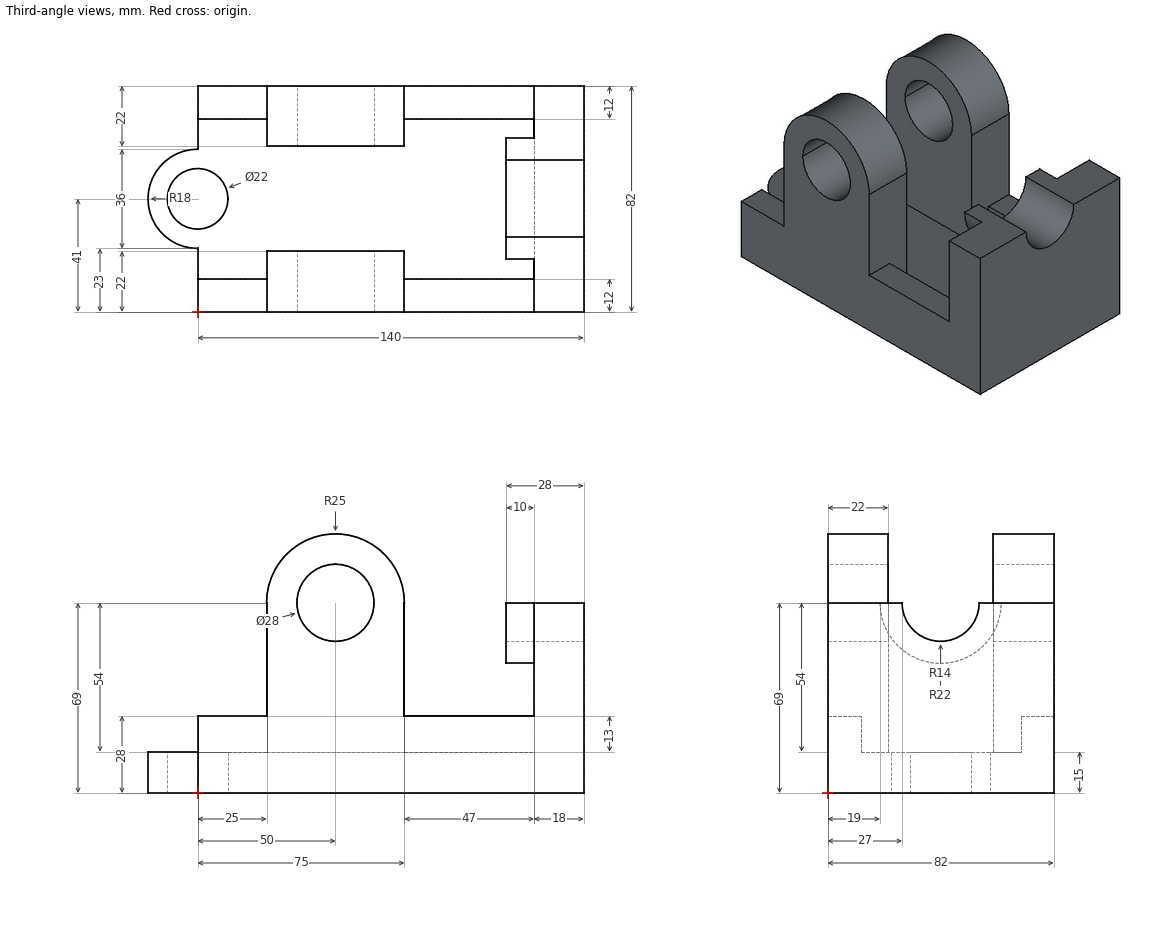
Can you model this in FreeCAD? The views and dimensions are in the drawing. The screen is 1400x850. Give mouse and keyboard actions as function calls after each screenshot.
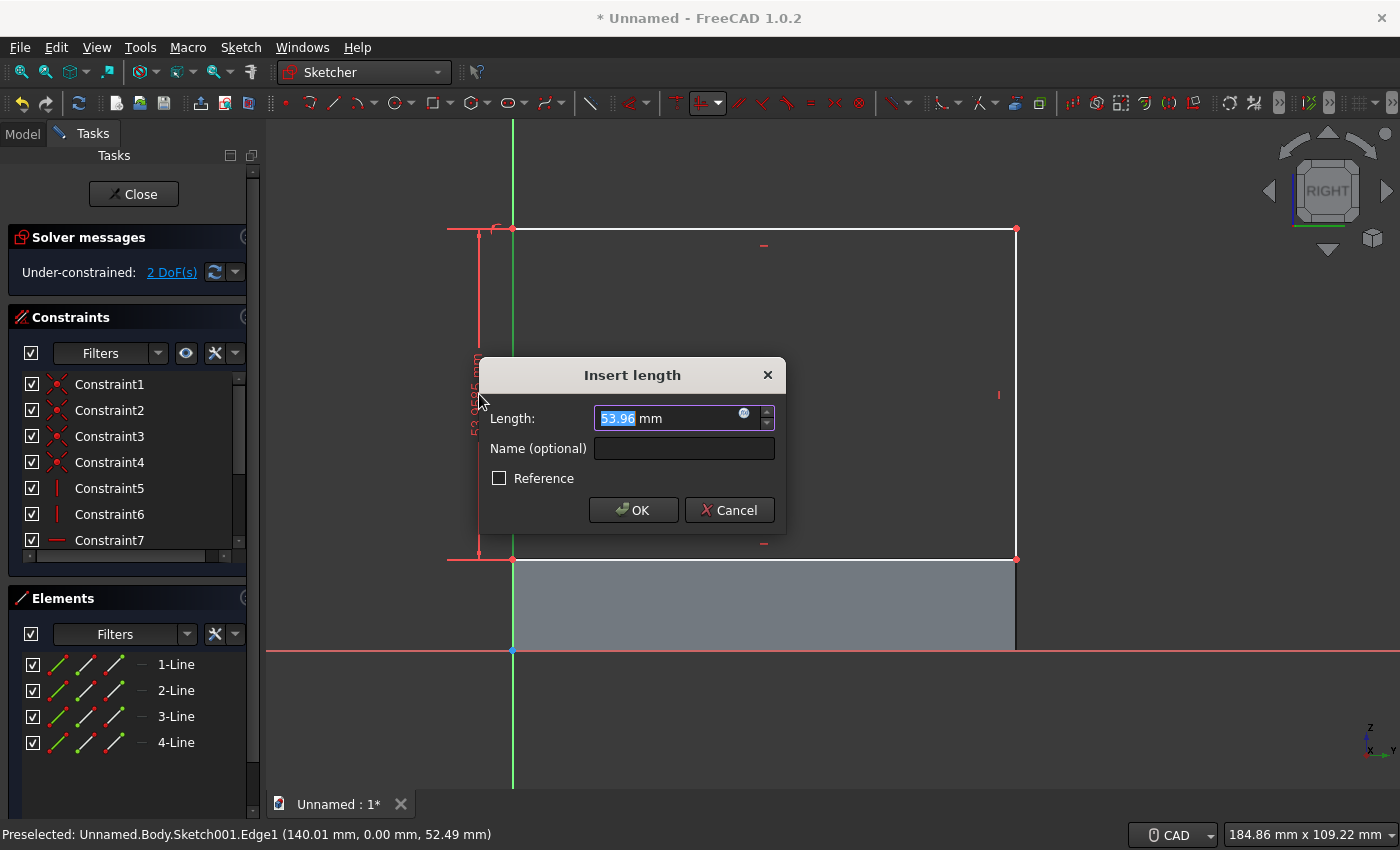
text(54)
key(Return)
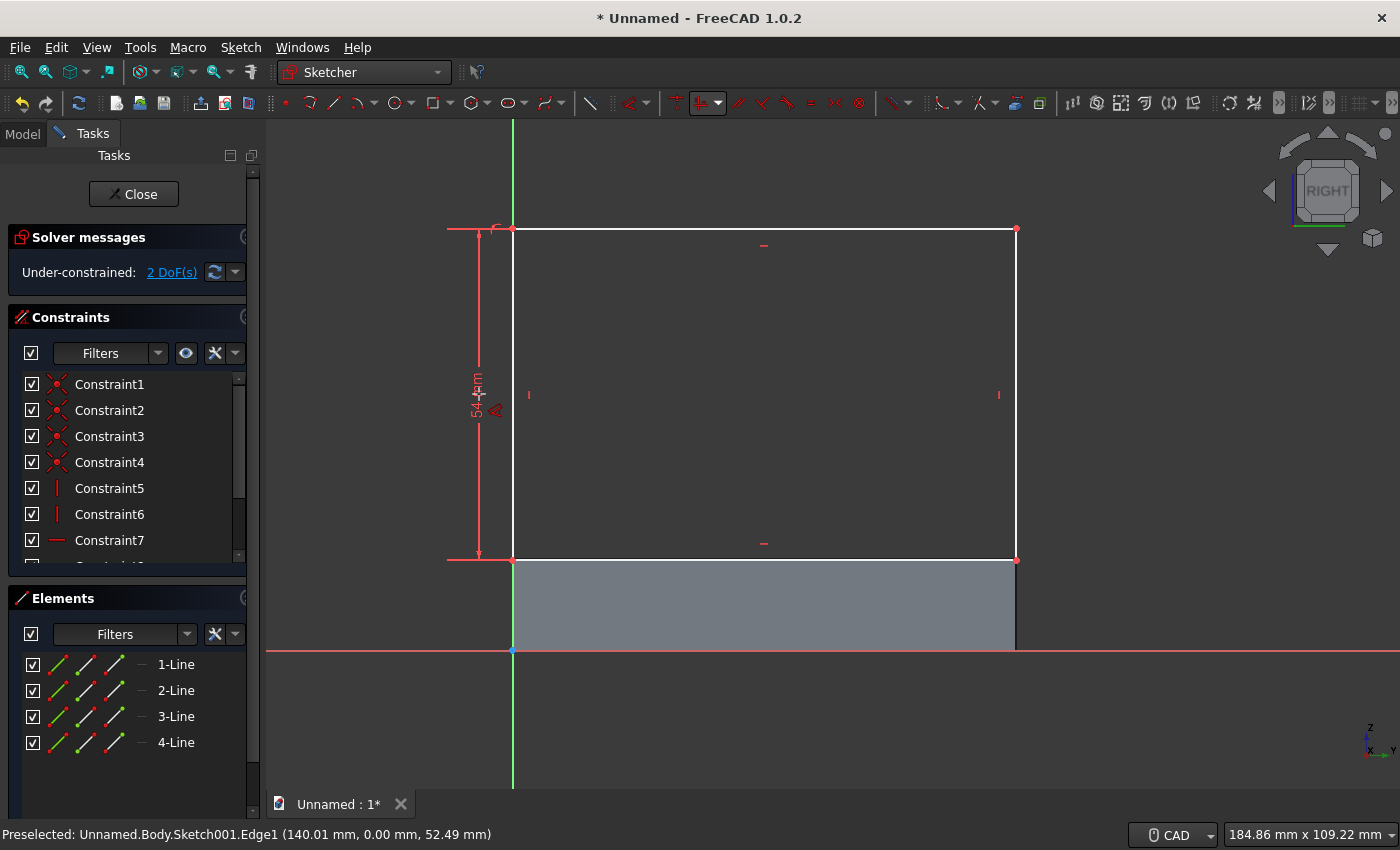
click(664, 560)
click(764, 594)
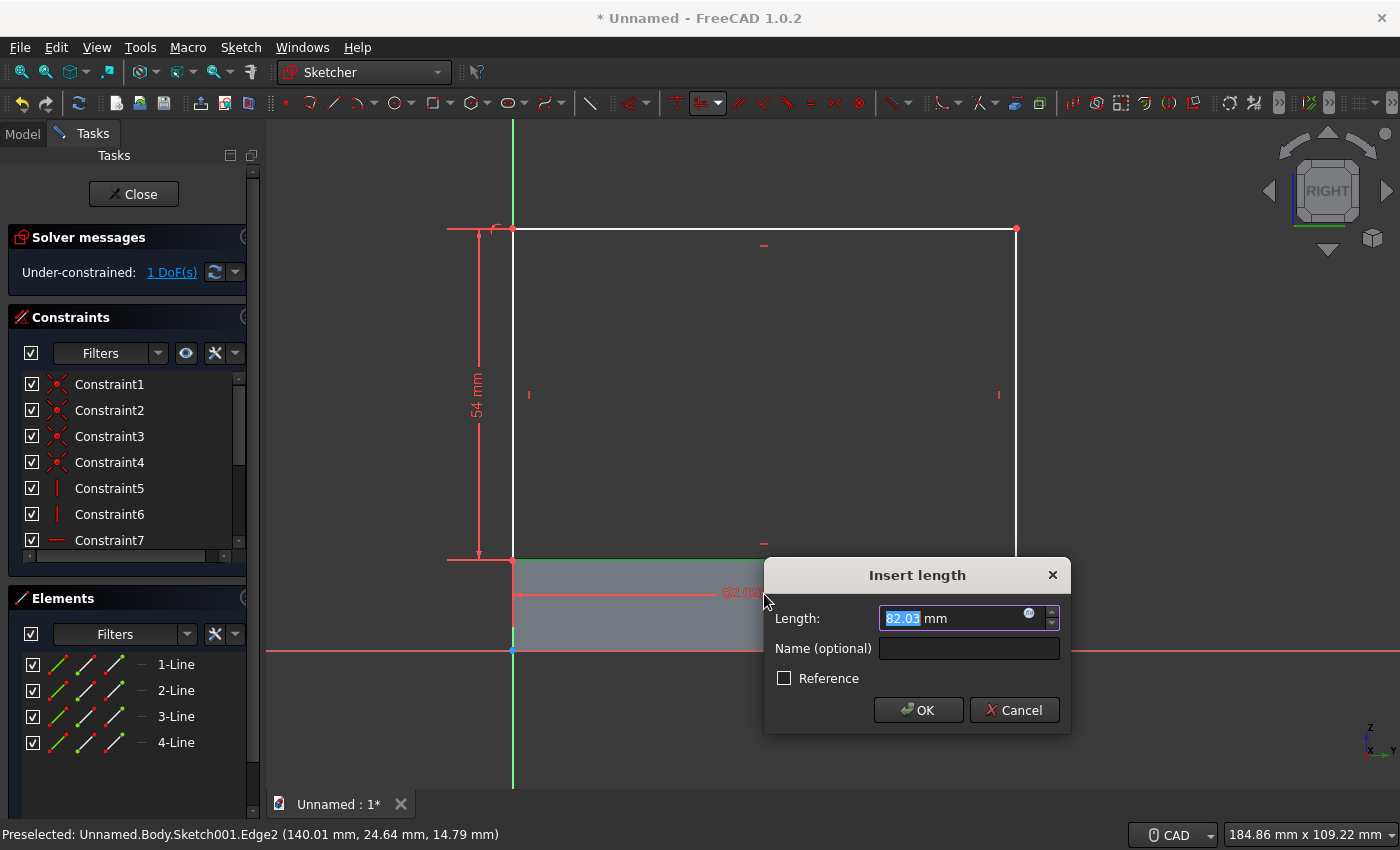
text(82)
key(Return)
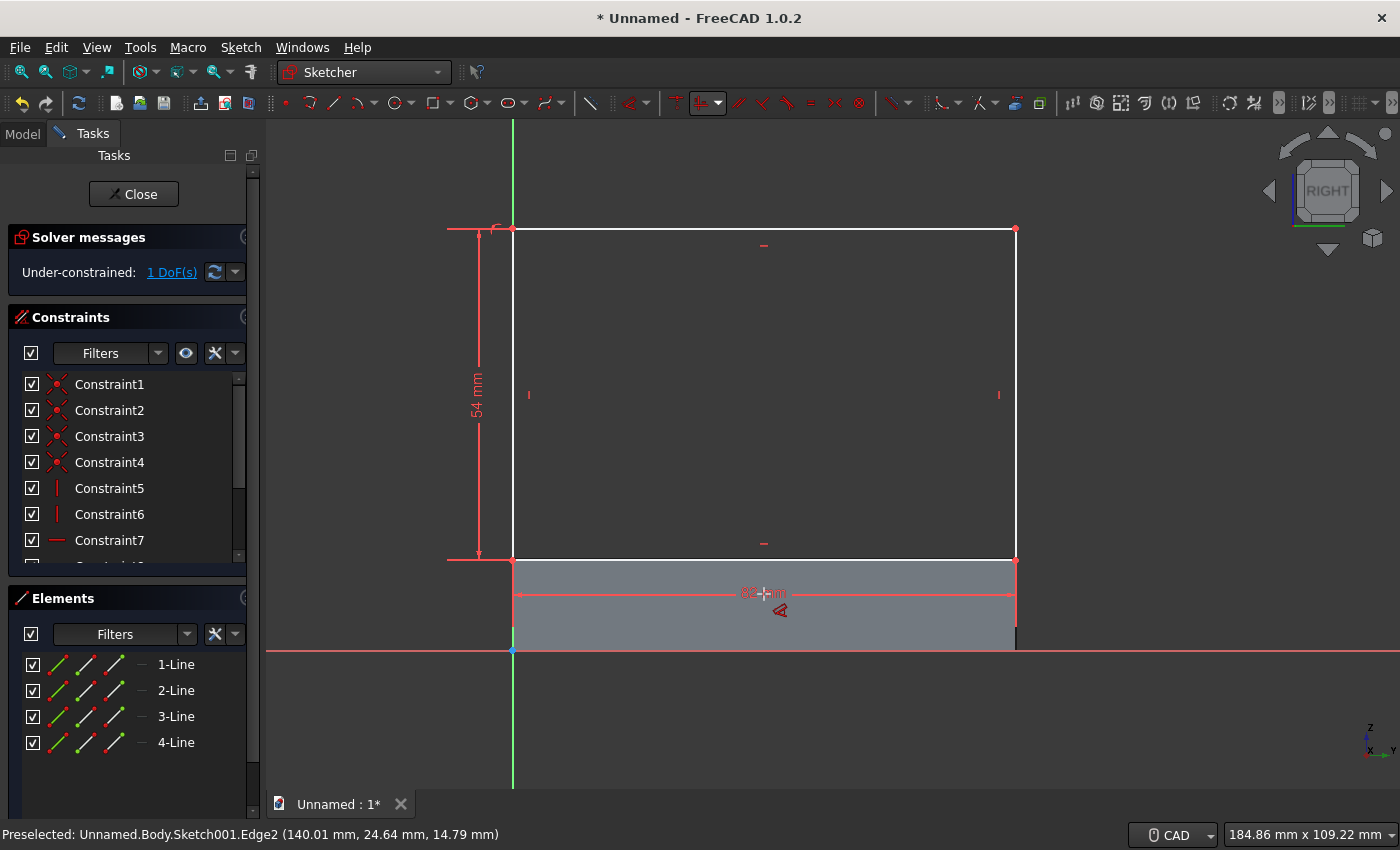
click(513, 229)
click(479, 440)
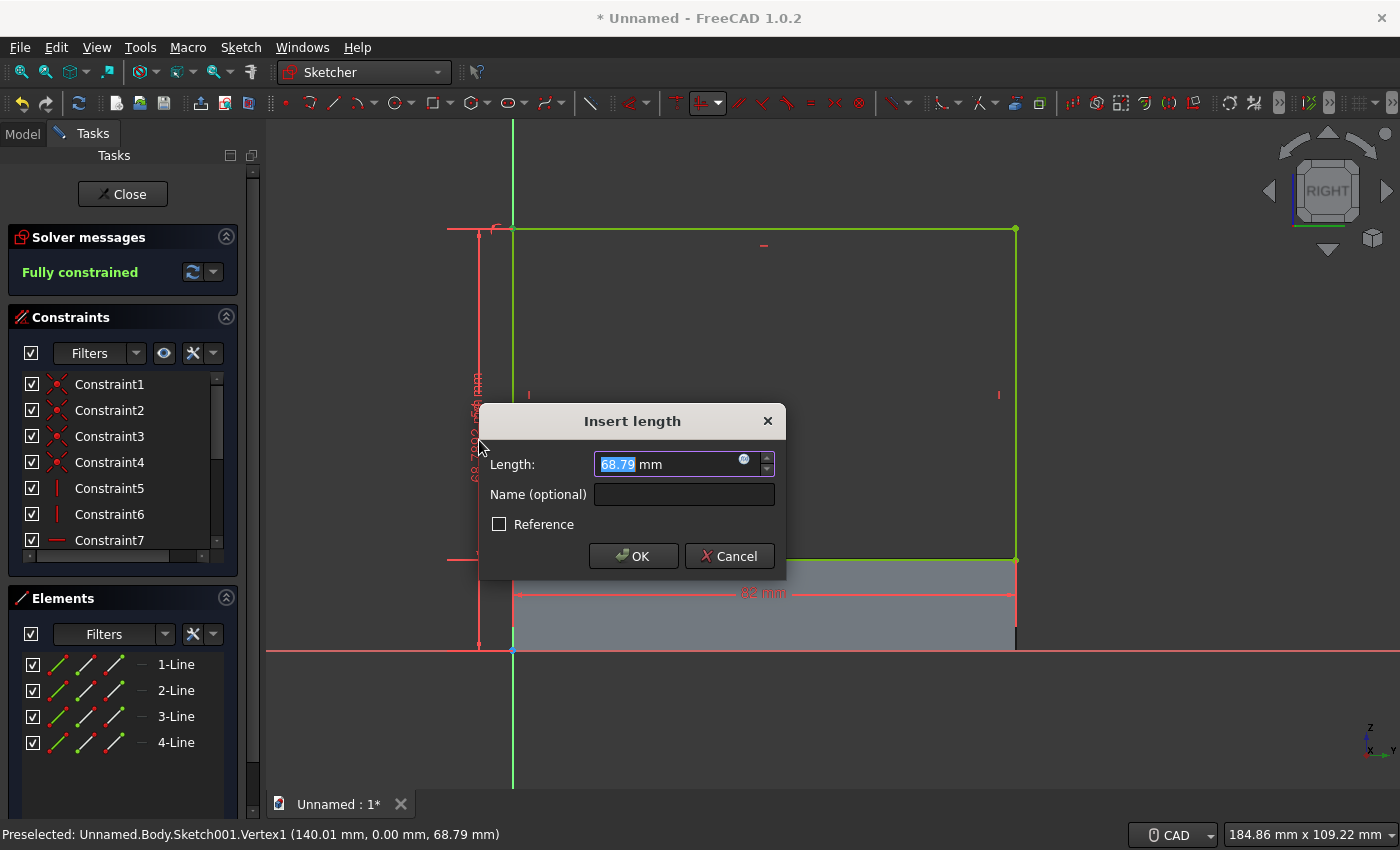
text(69)
key(Return)
key(Escape)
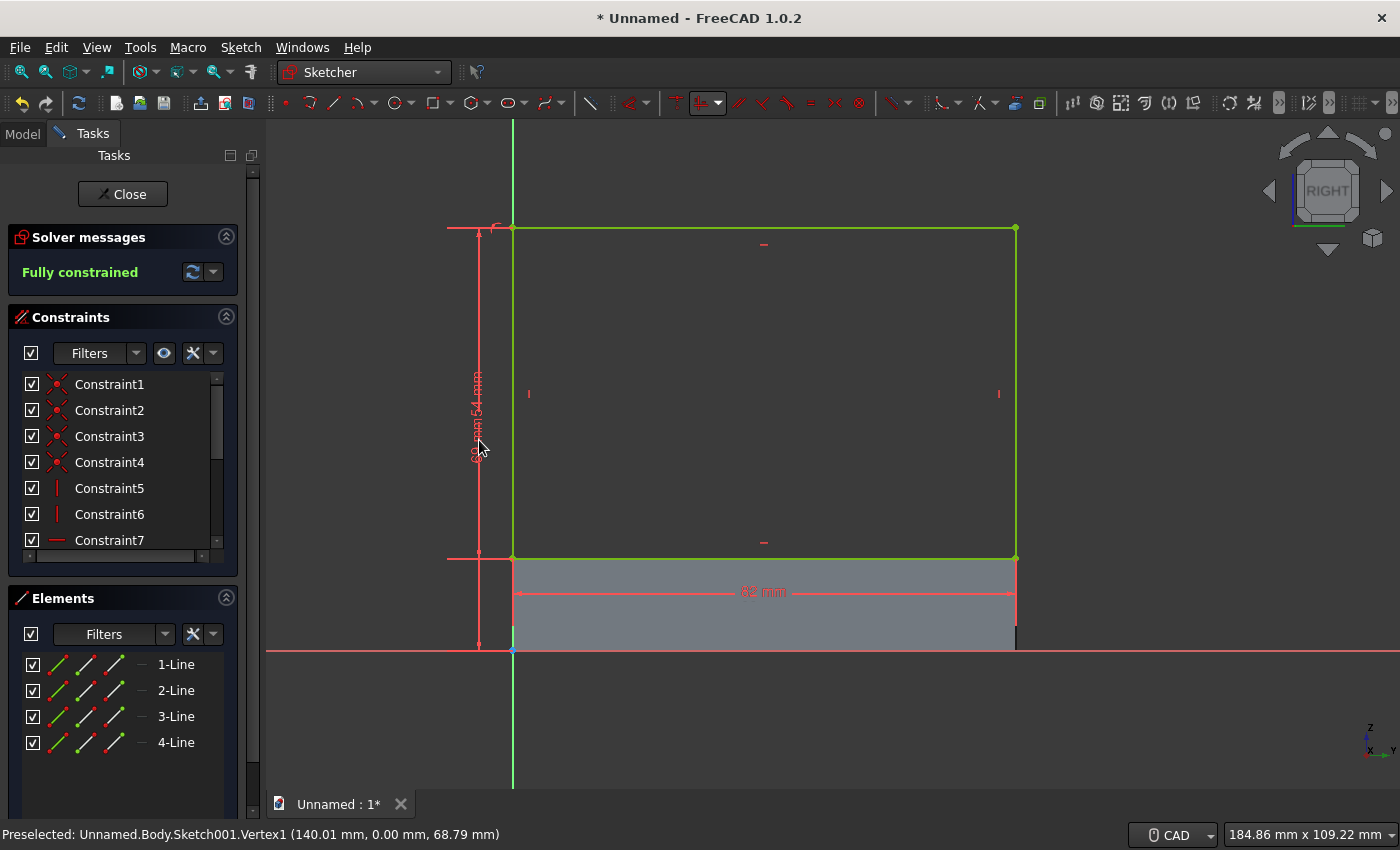
click(123, 194)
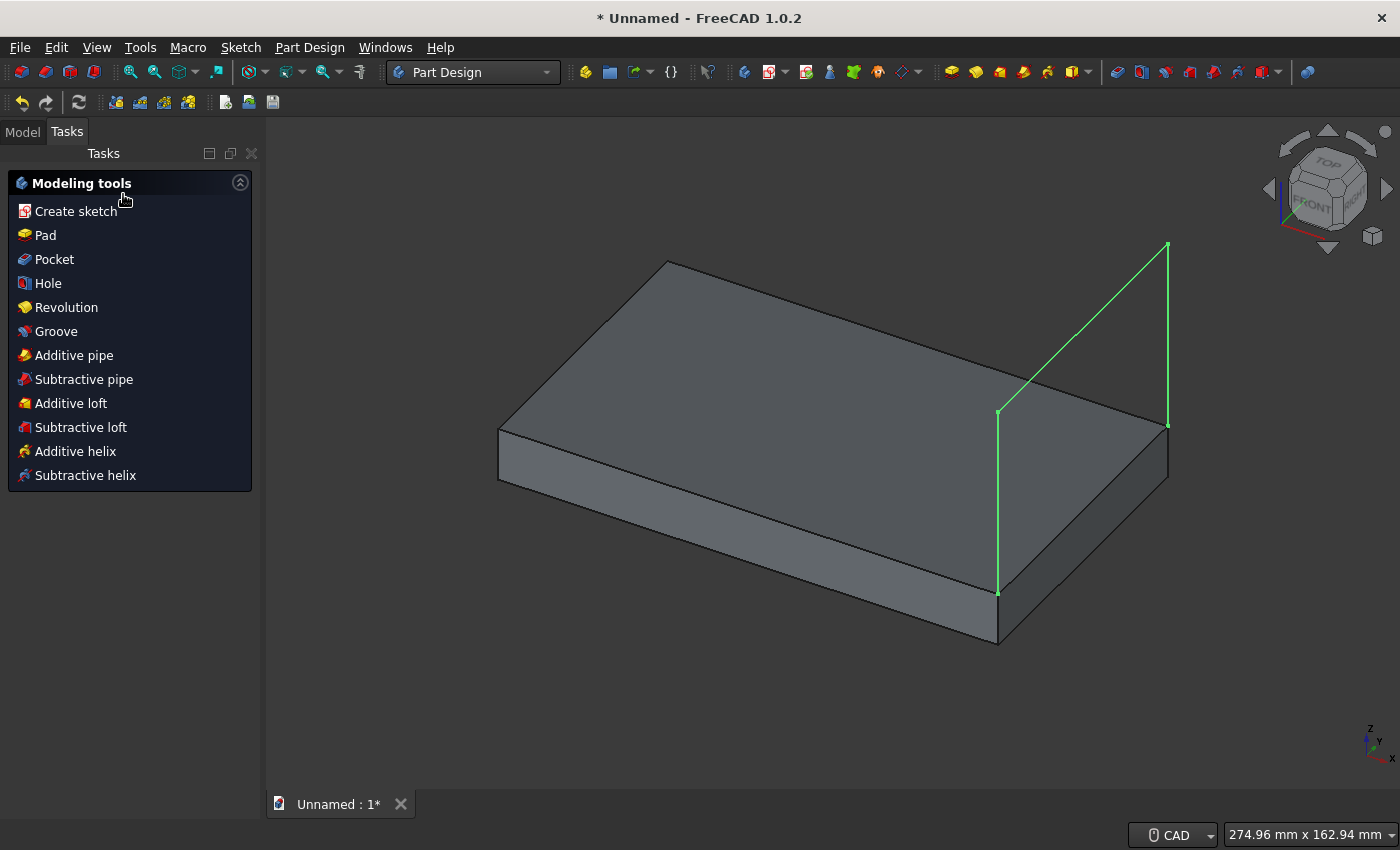
click(952, 72)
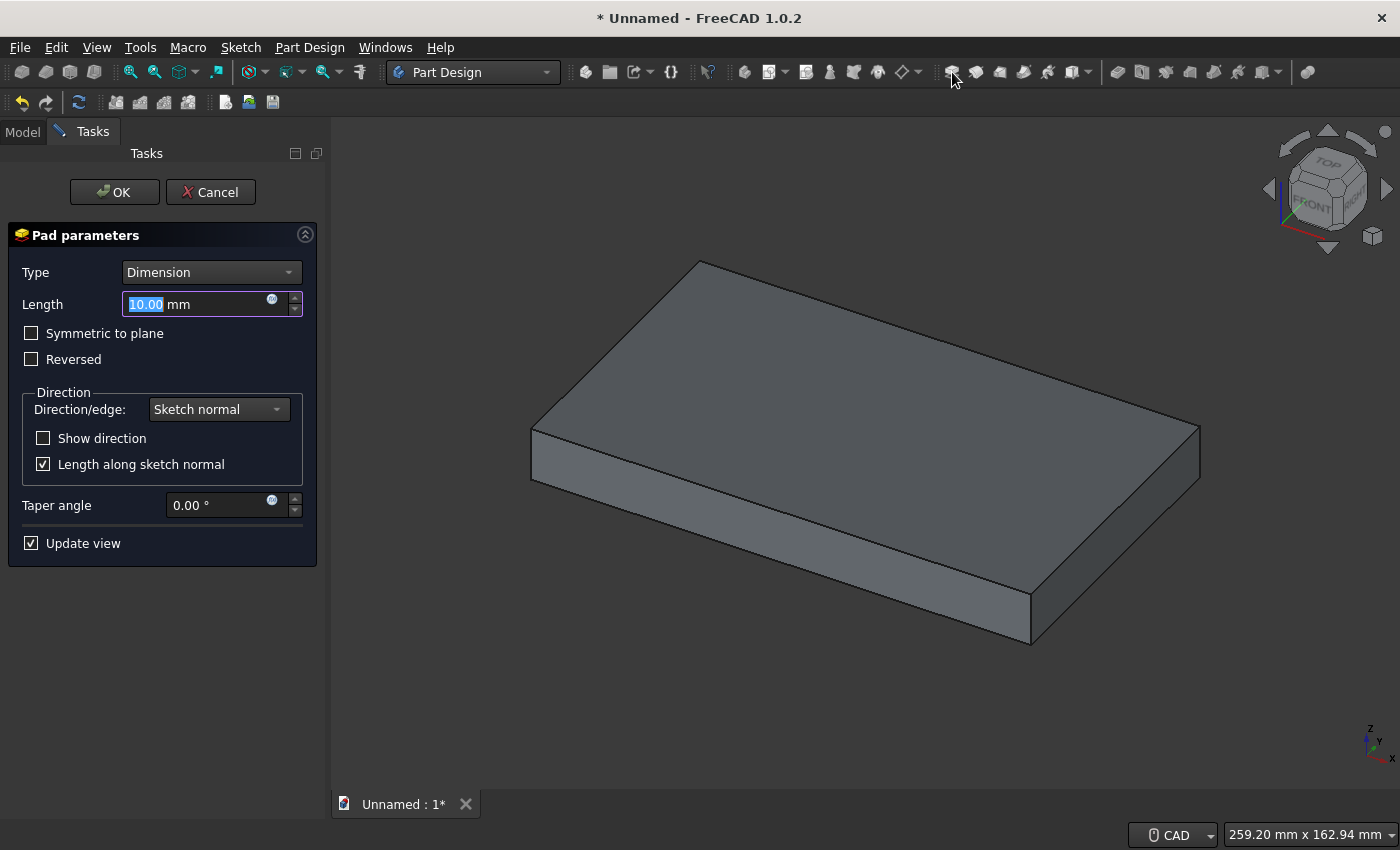
text(18)
key(Tab)